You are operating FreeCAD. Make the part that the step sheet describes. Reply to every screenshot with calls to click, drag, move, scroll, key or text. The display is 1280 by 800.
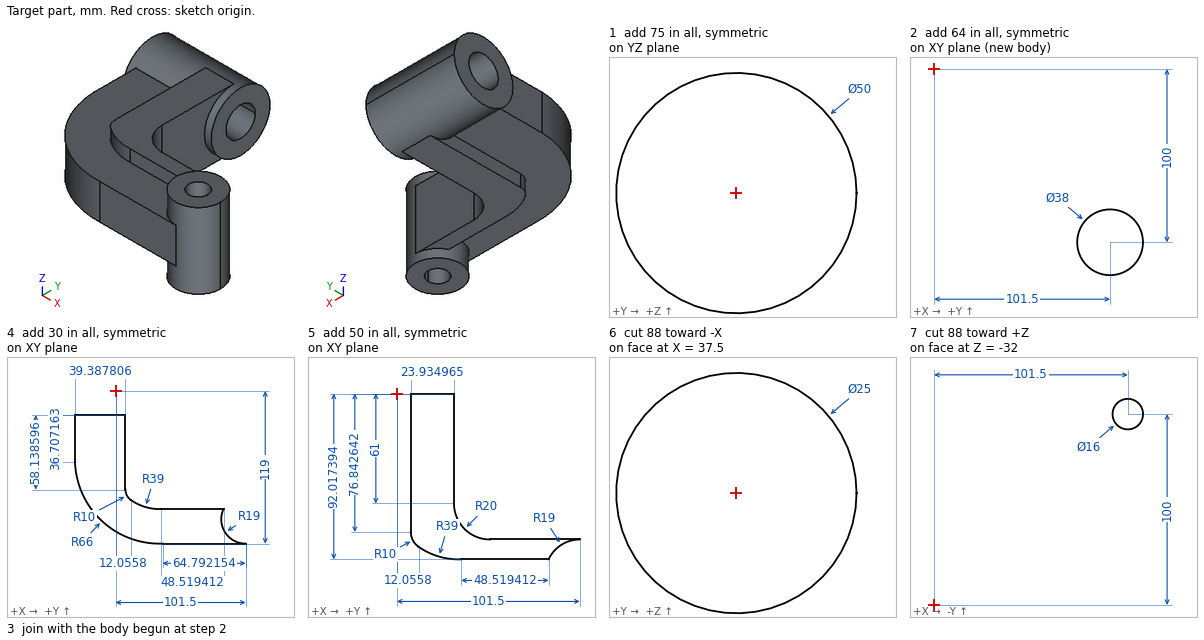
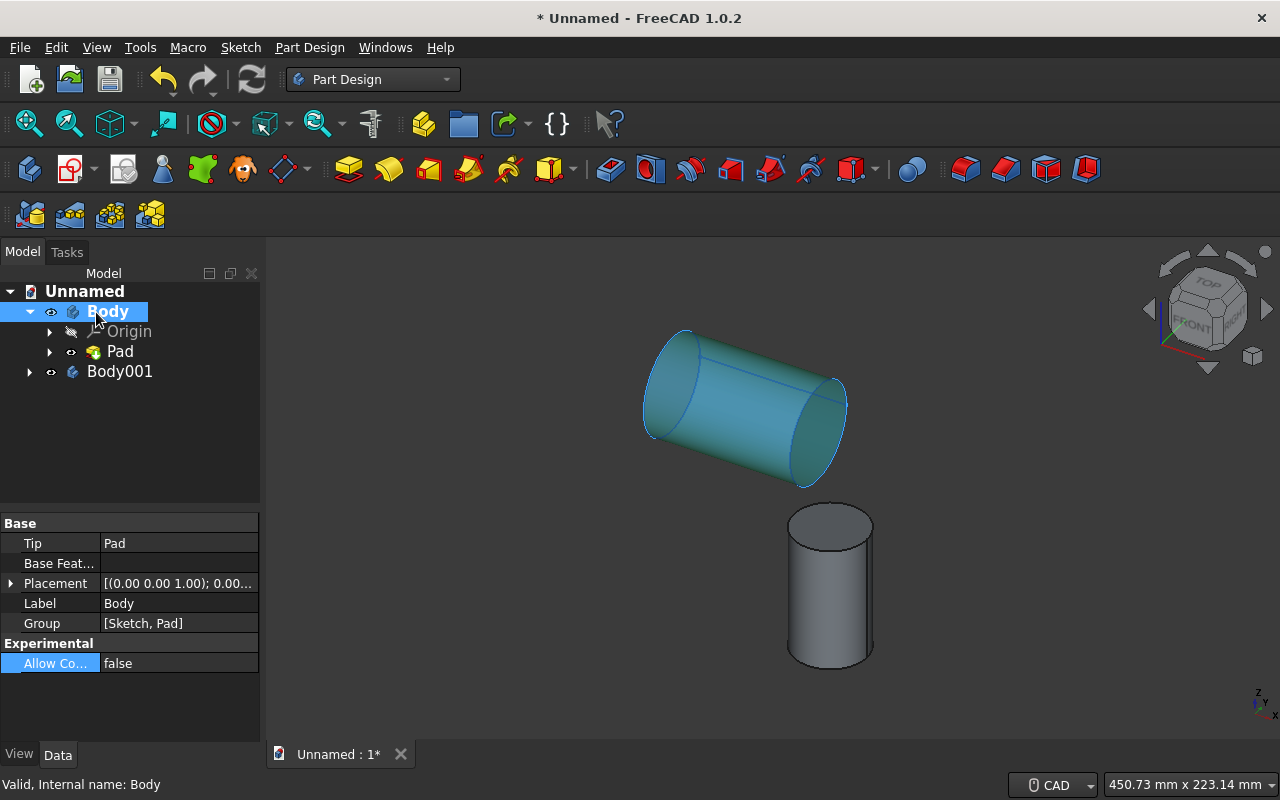
click(146, 663)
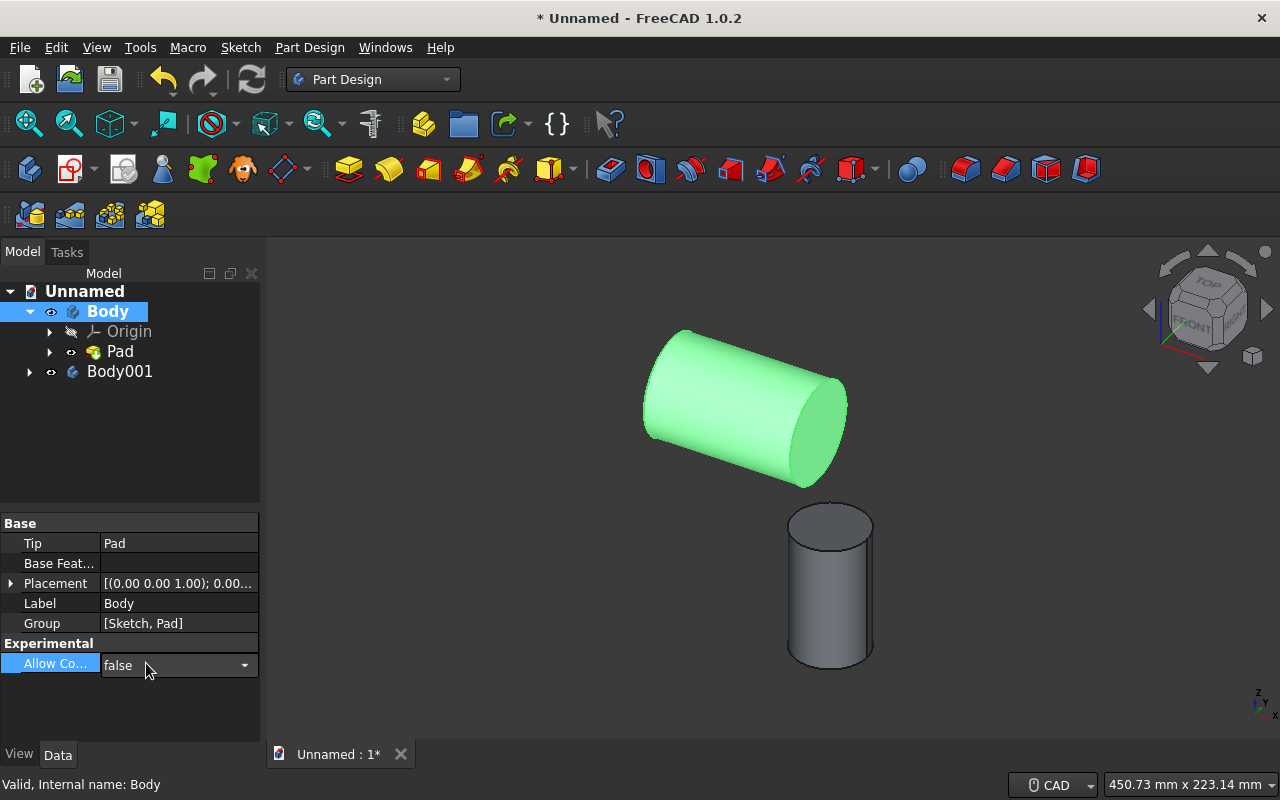
click(146, 663)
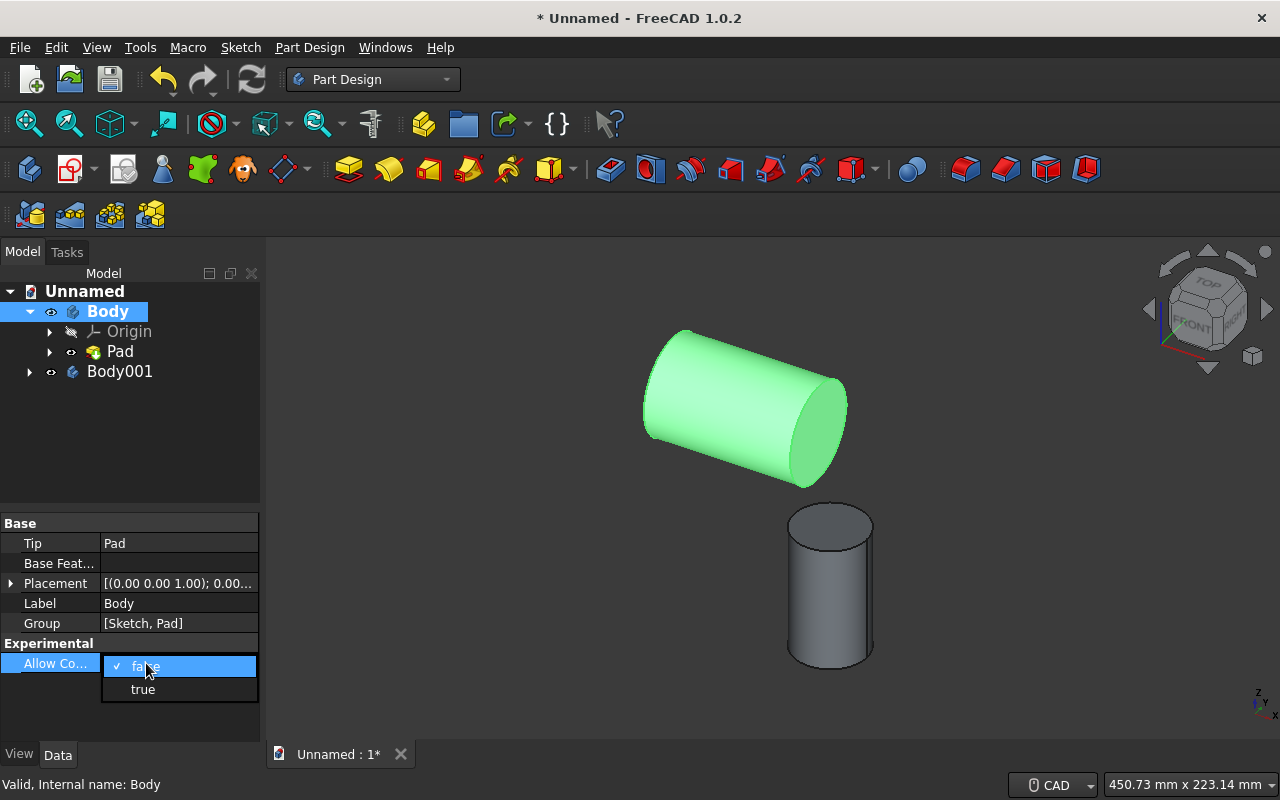
click(179, 690)
key(Return)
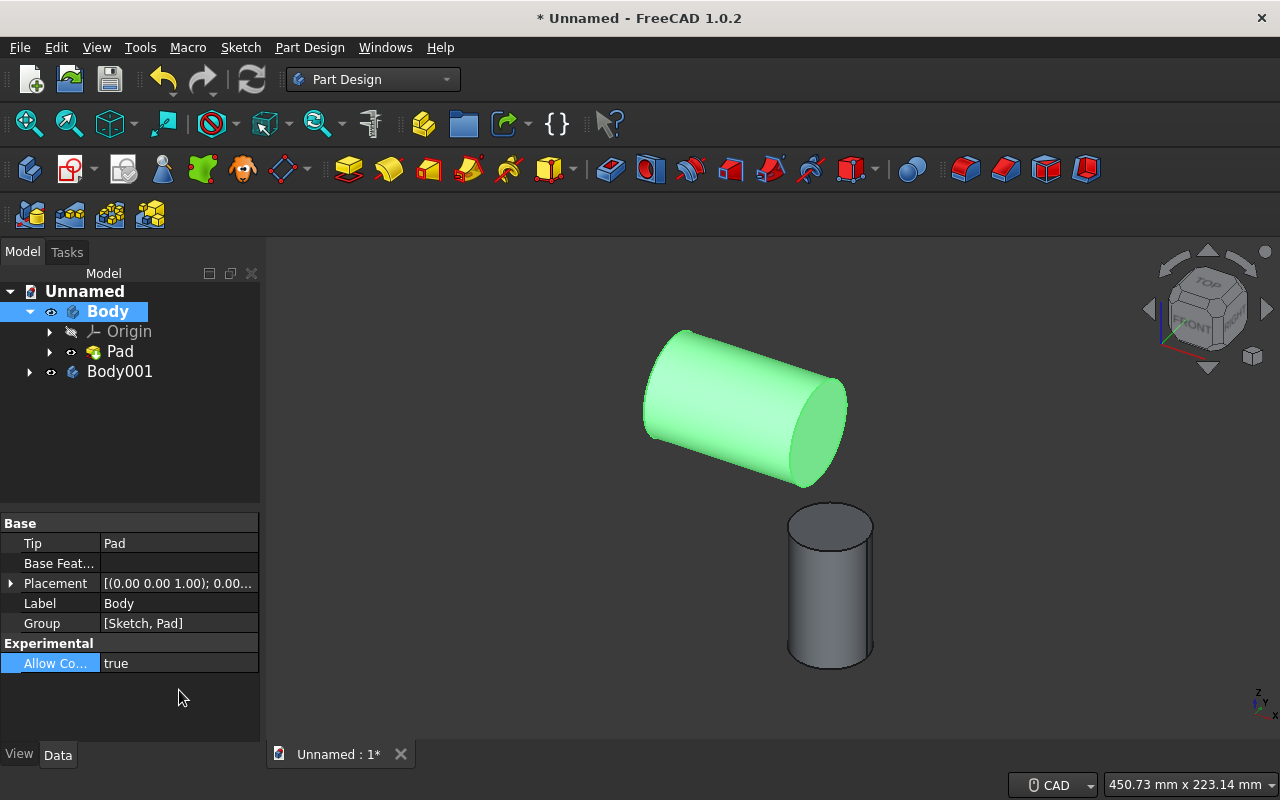
click(96, 372)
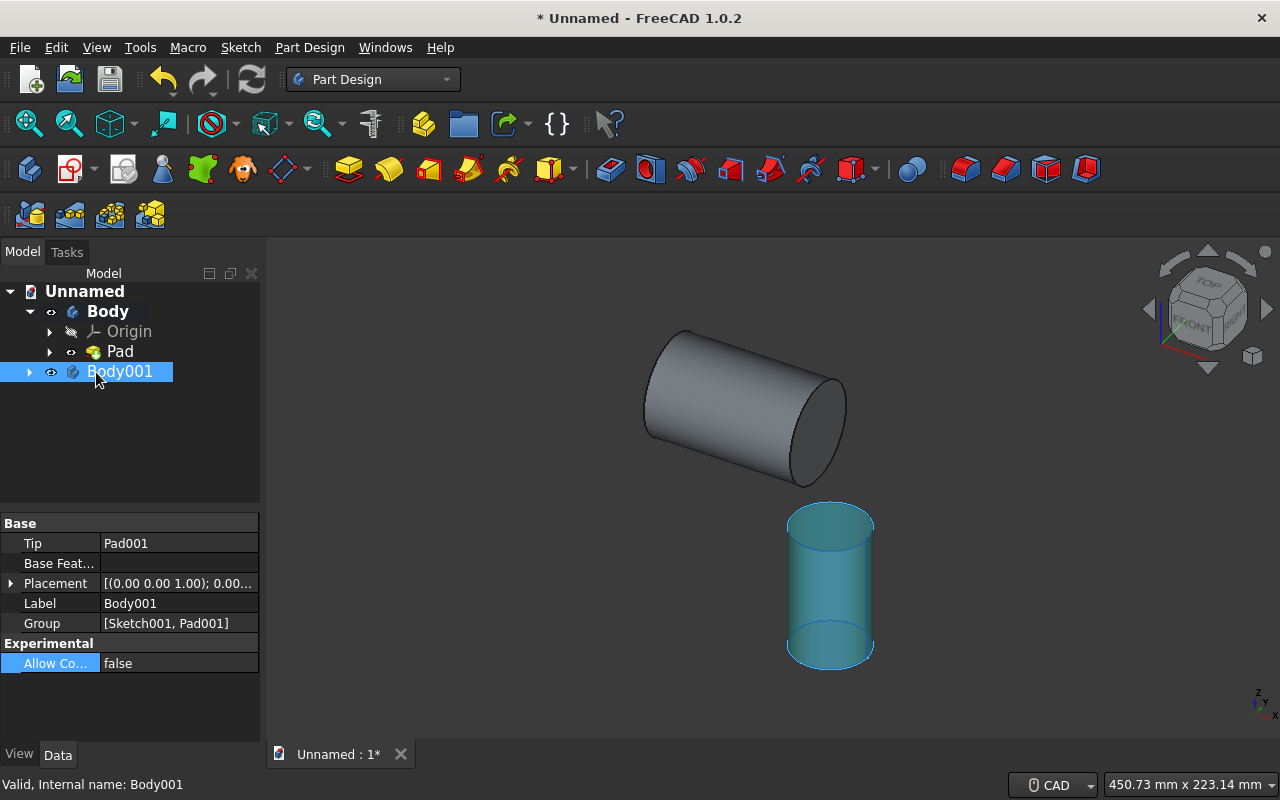
click(914, 170)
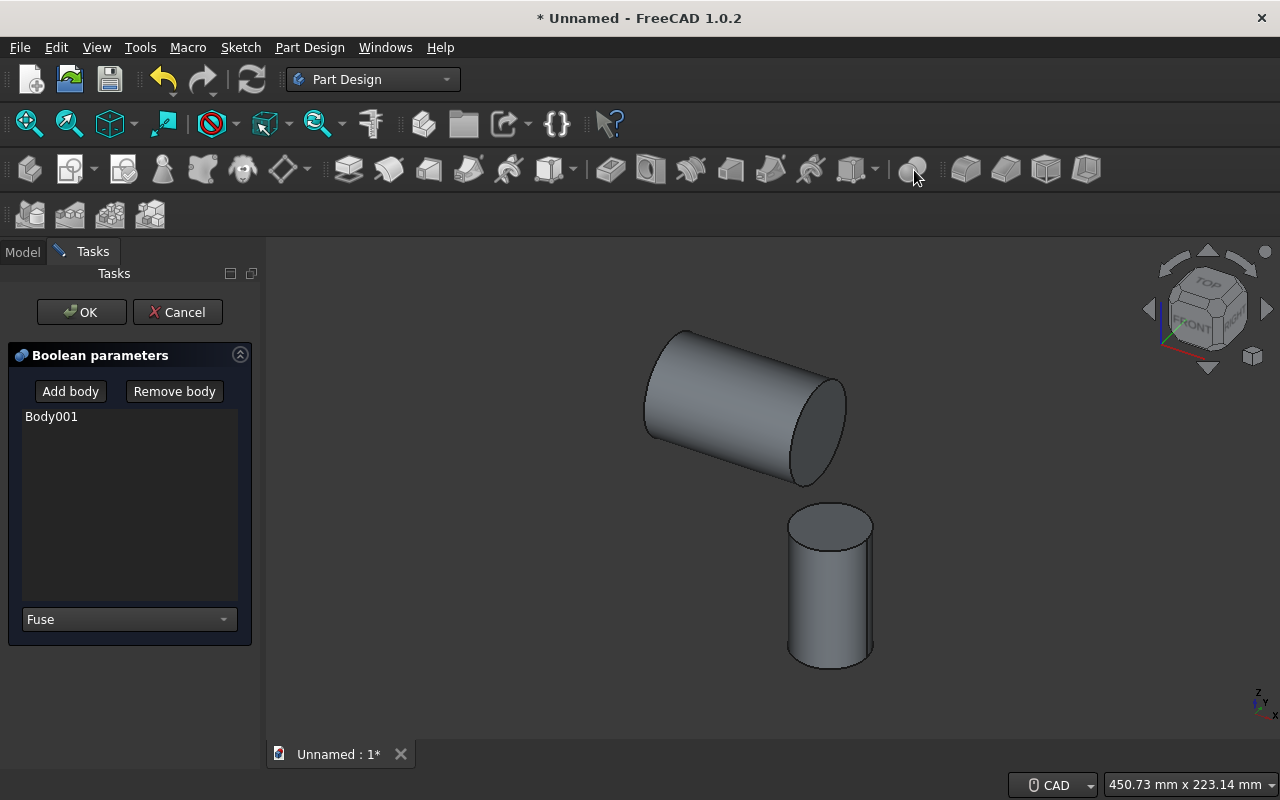
click(82, 312)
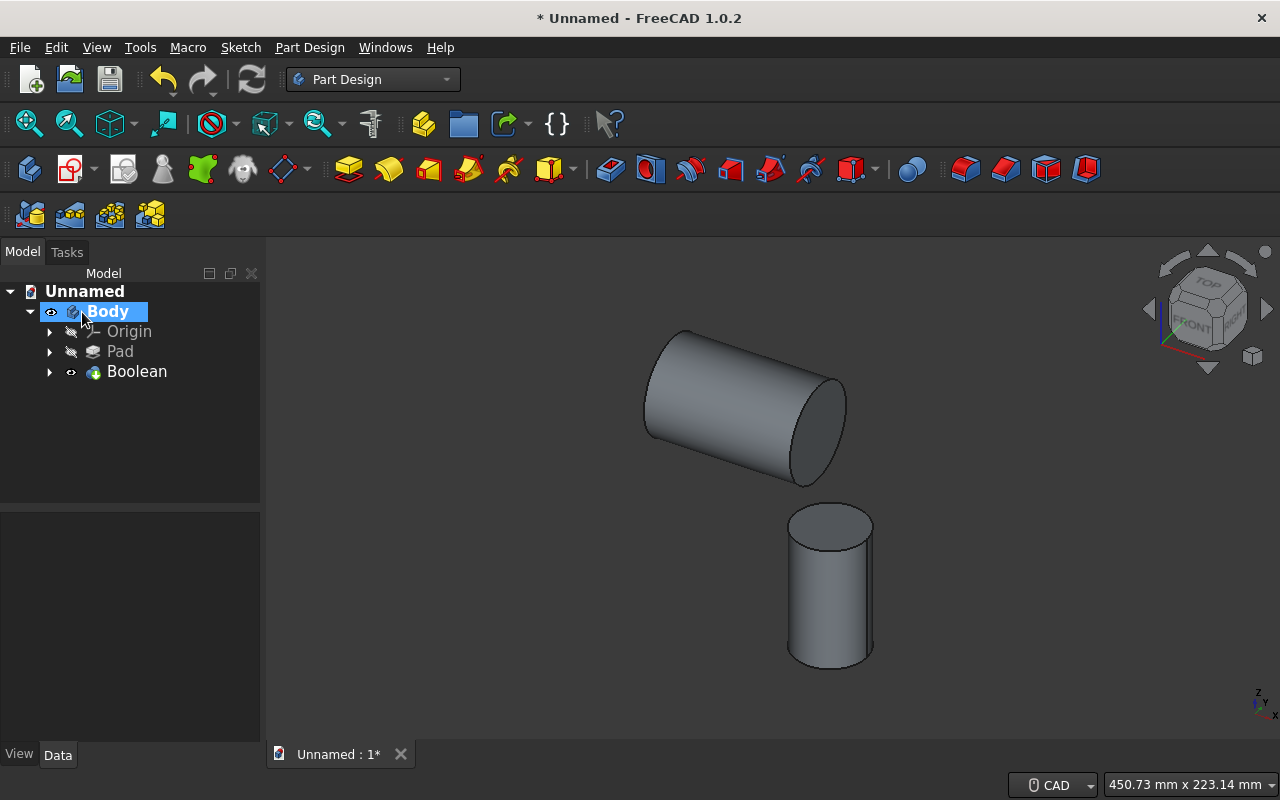
click(70, 170)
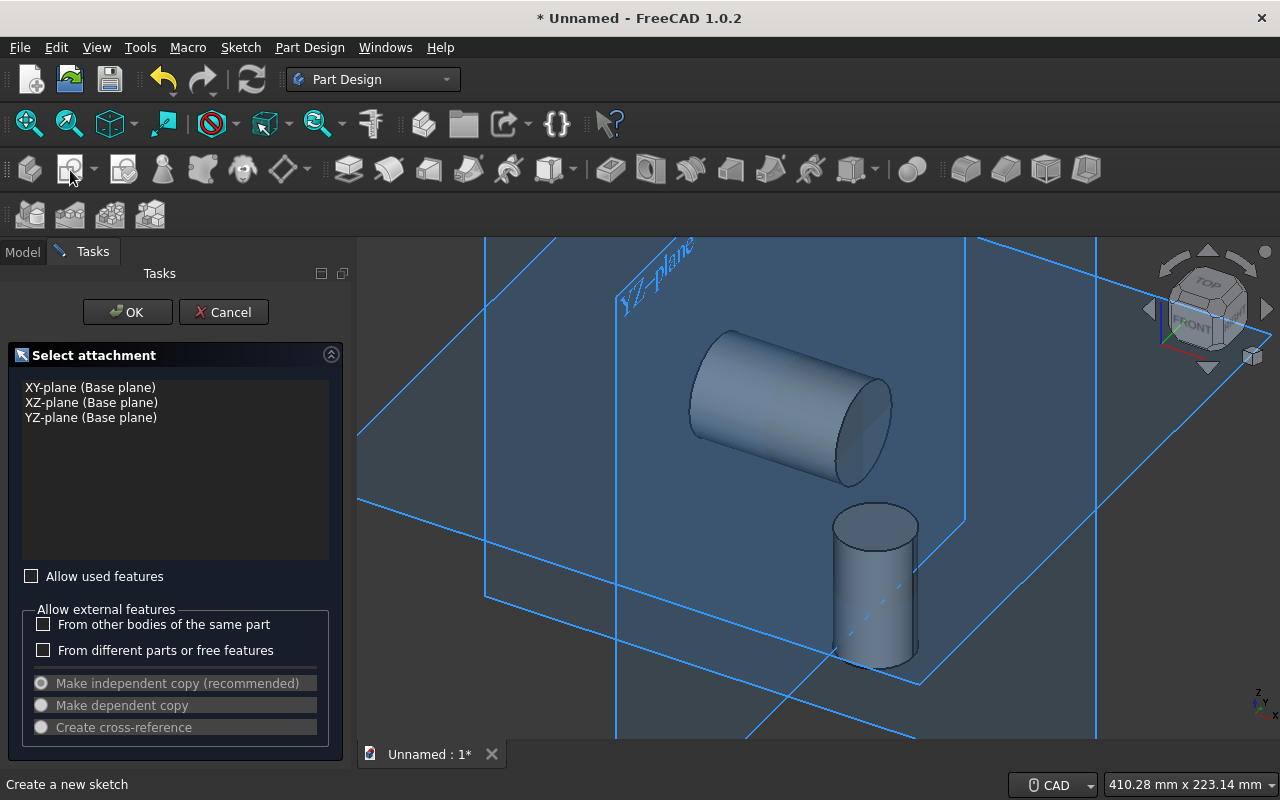
click(82, 388)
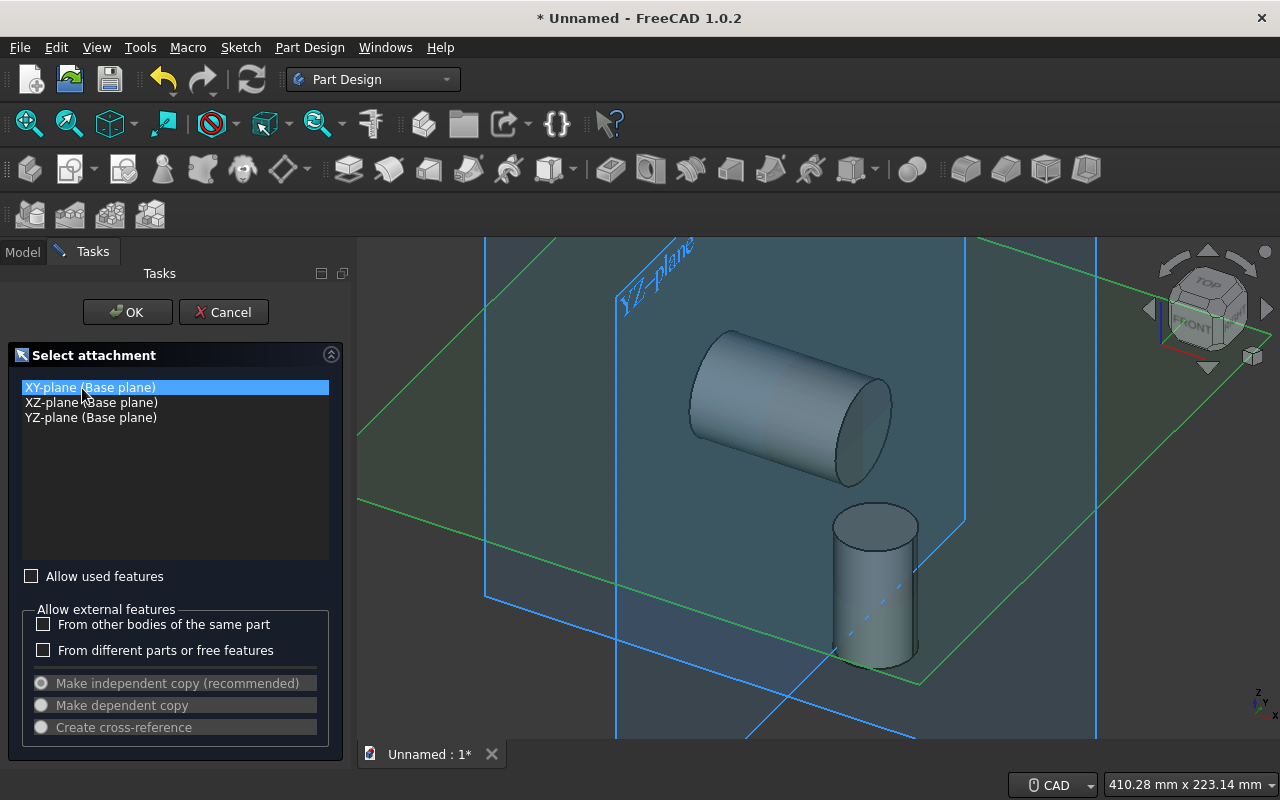
click(128, 312)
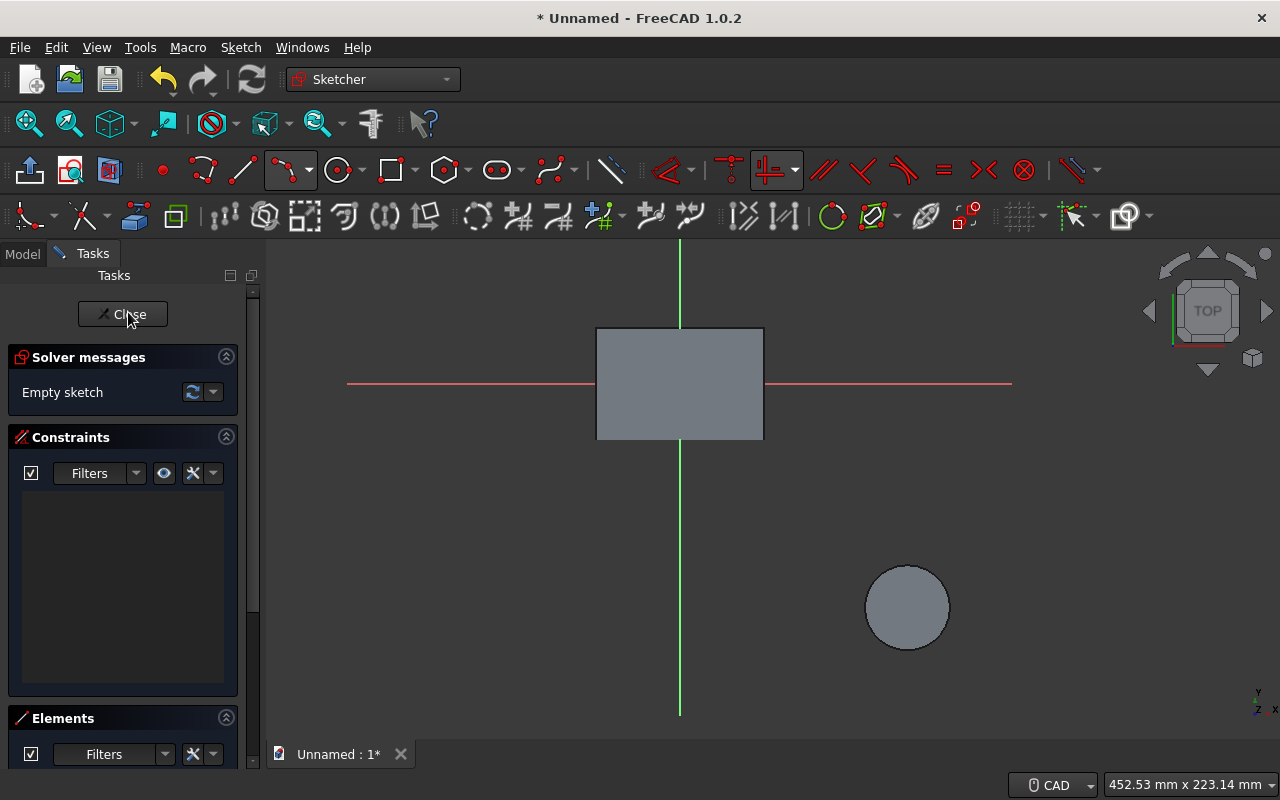
click(110, 170)